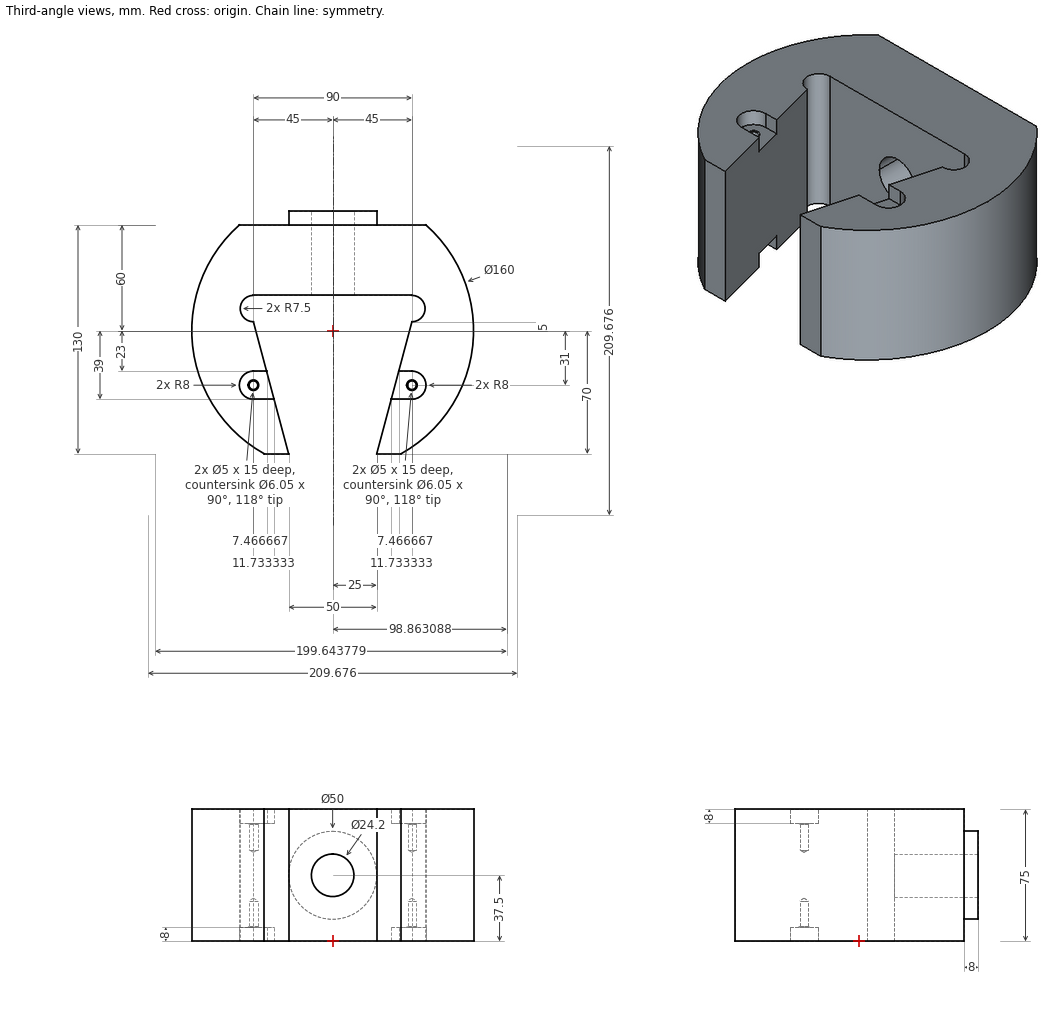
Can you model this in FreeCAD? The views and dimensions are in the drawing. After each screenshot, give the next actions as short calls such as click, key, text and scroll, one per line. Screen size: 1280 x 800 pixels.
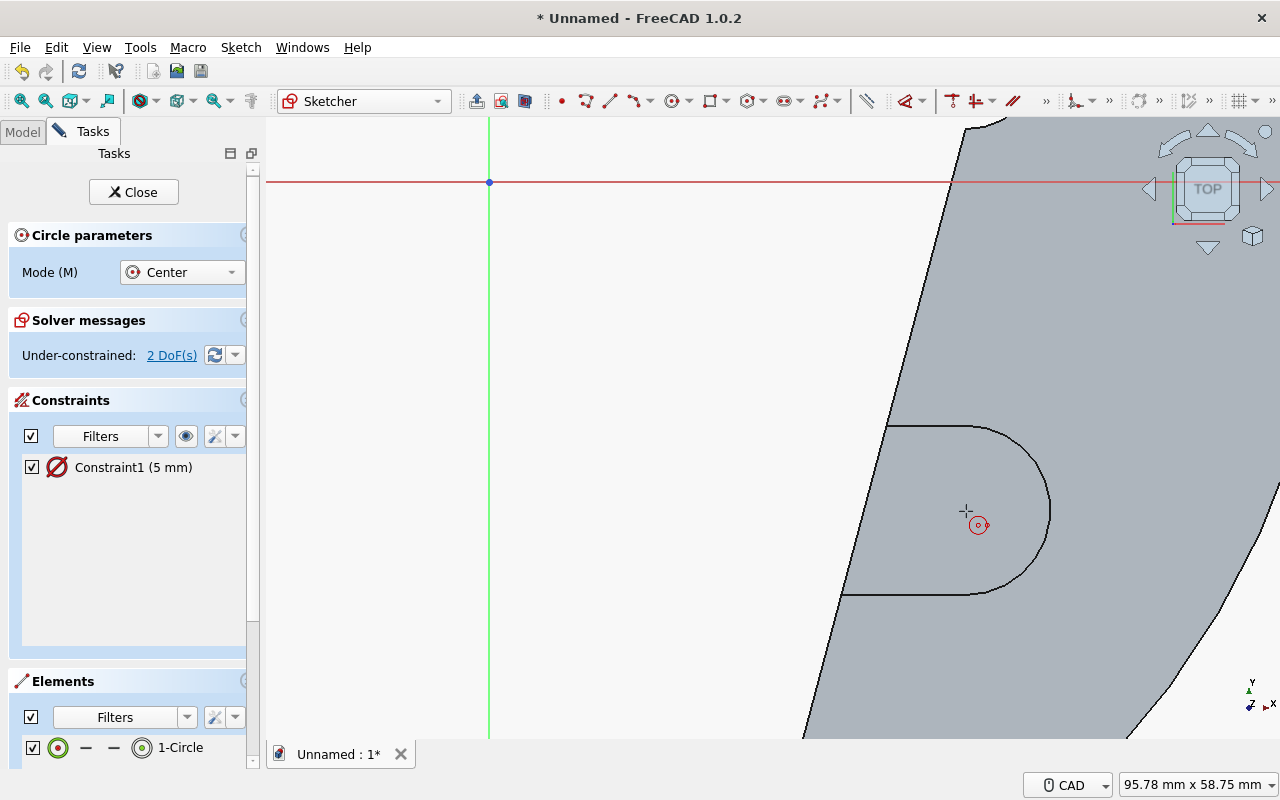
click(966, 510)
move(984, 492)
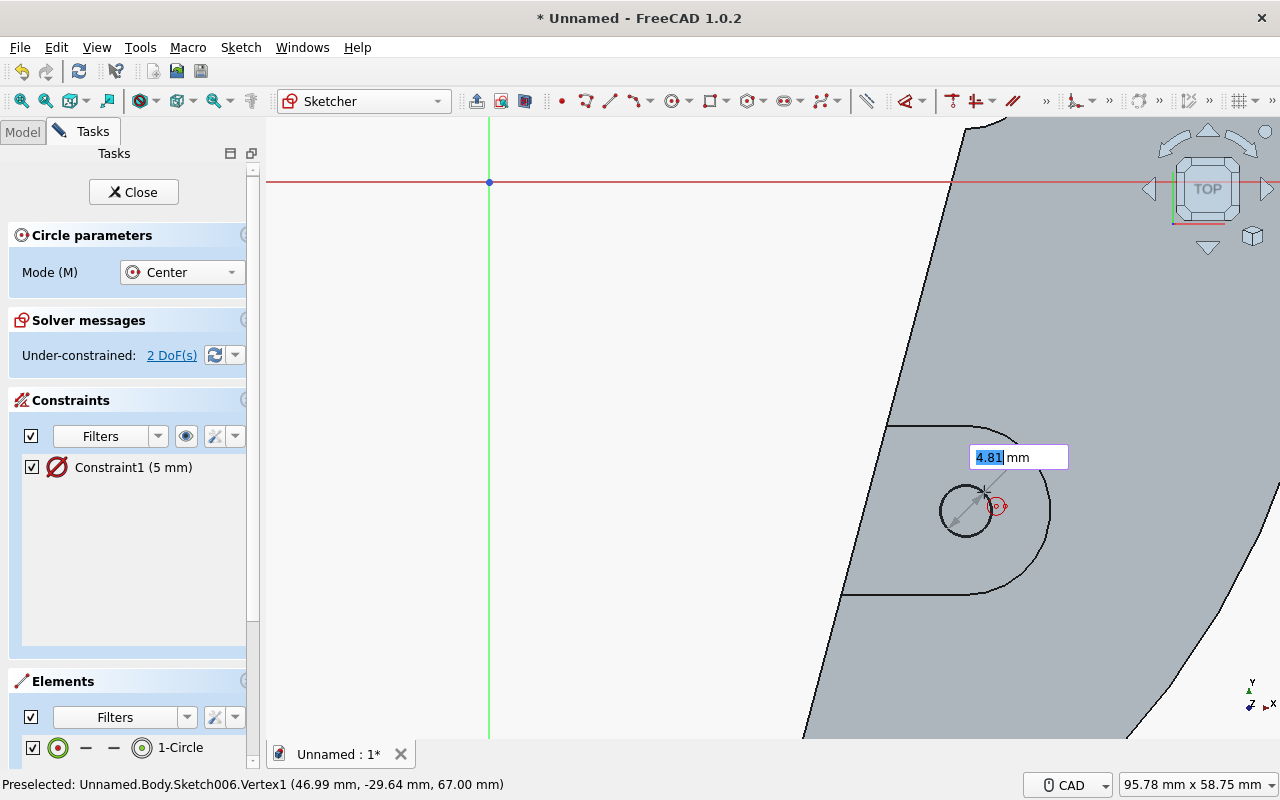
text(5)
key(Return)
key(Escape)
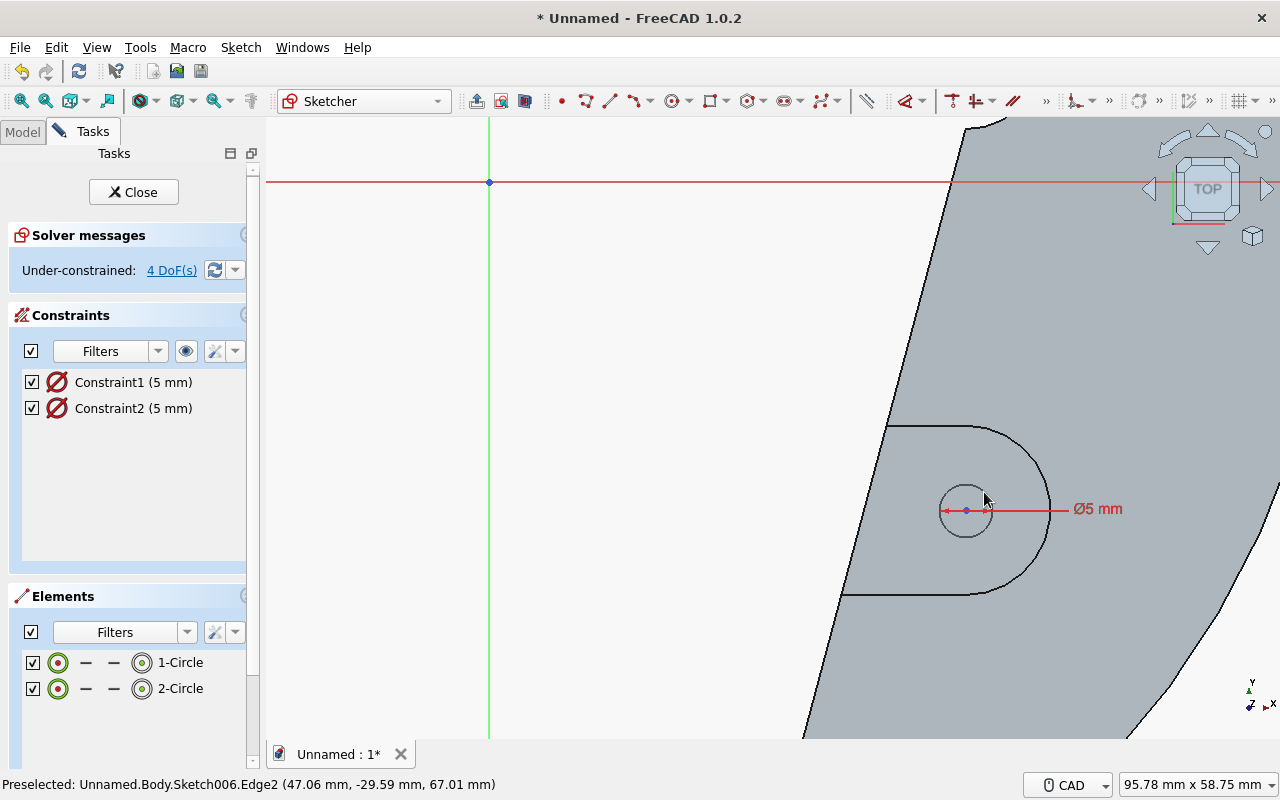
scroll(966, 511, down, 3)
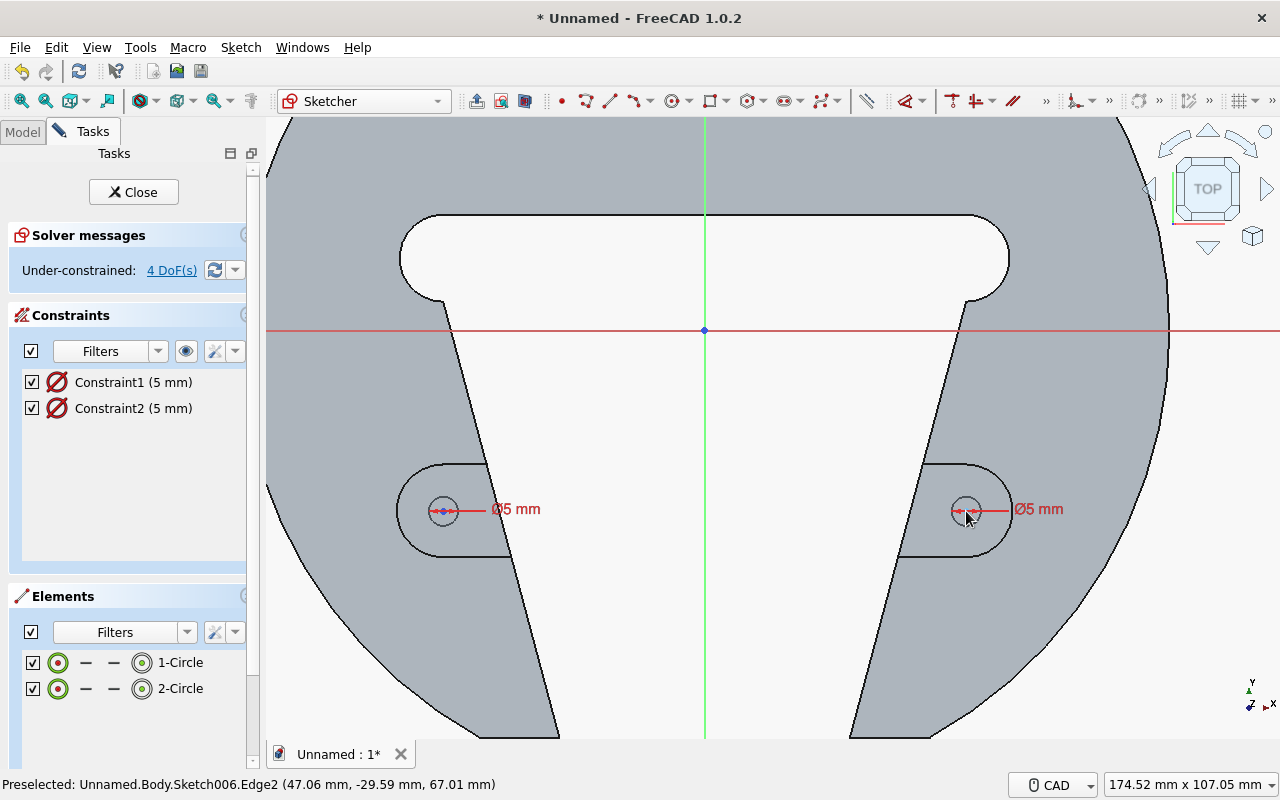
click(443, 511)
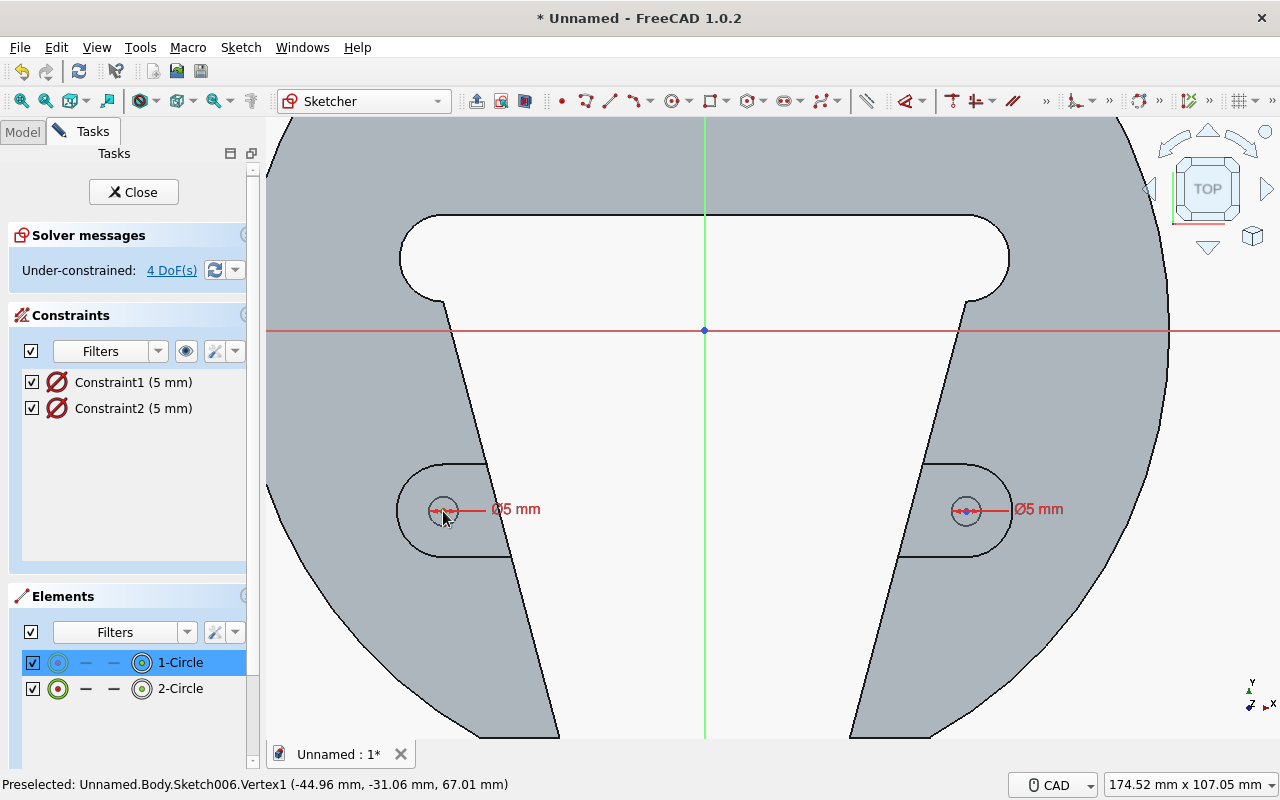
click(966, 511)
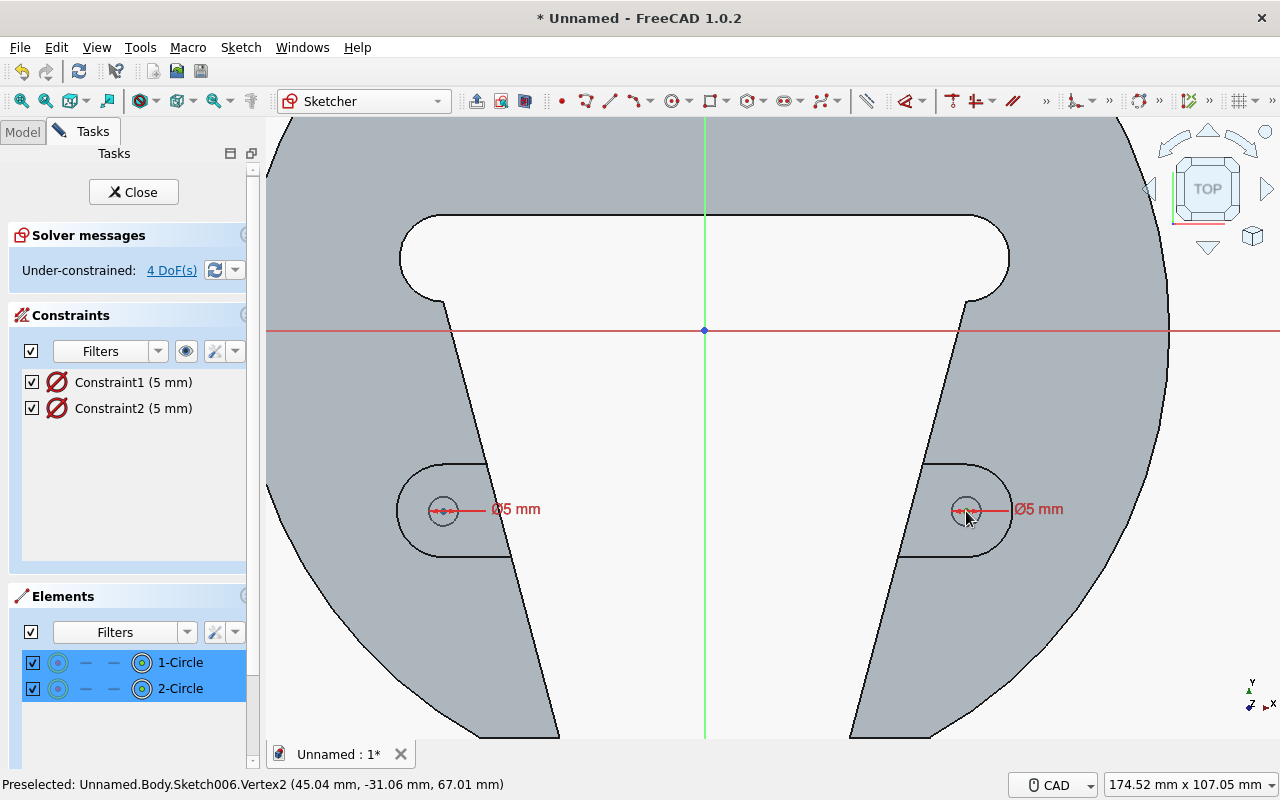
key(h)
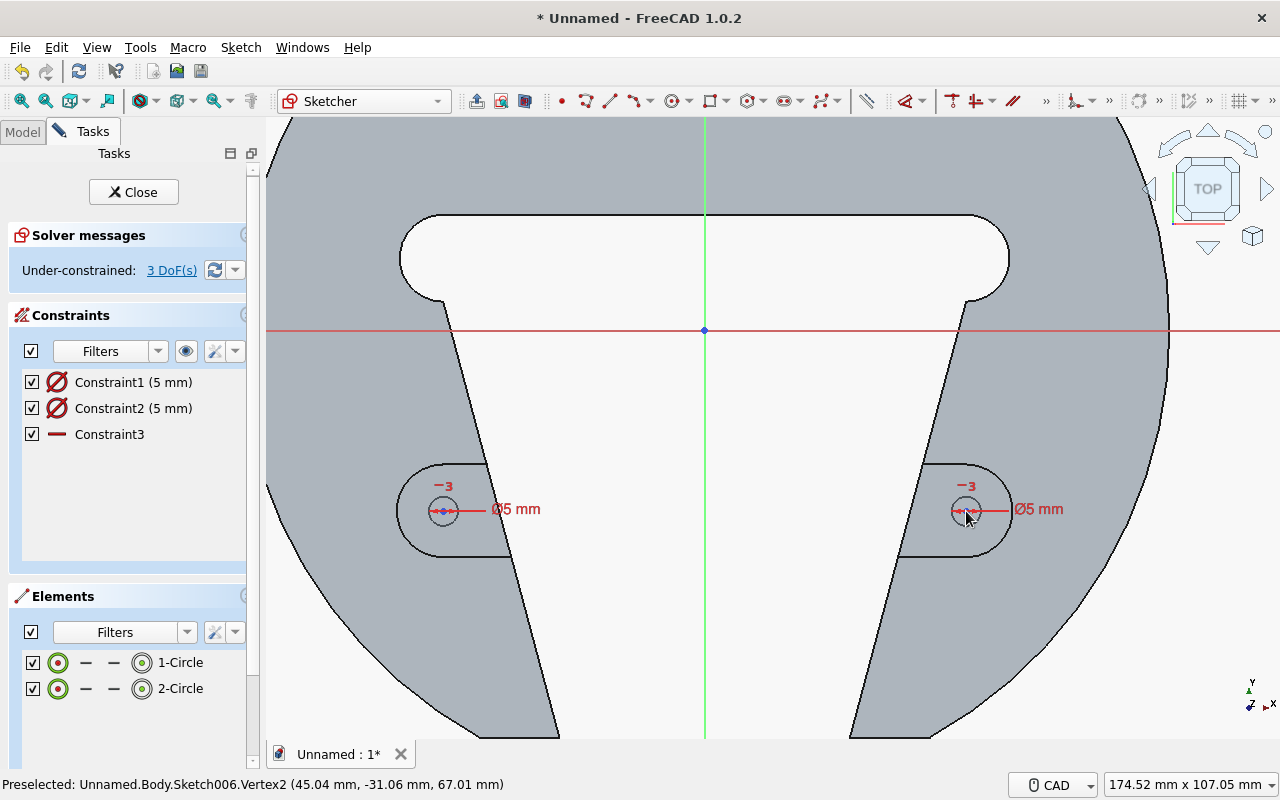
key(d)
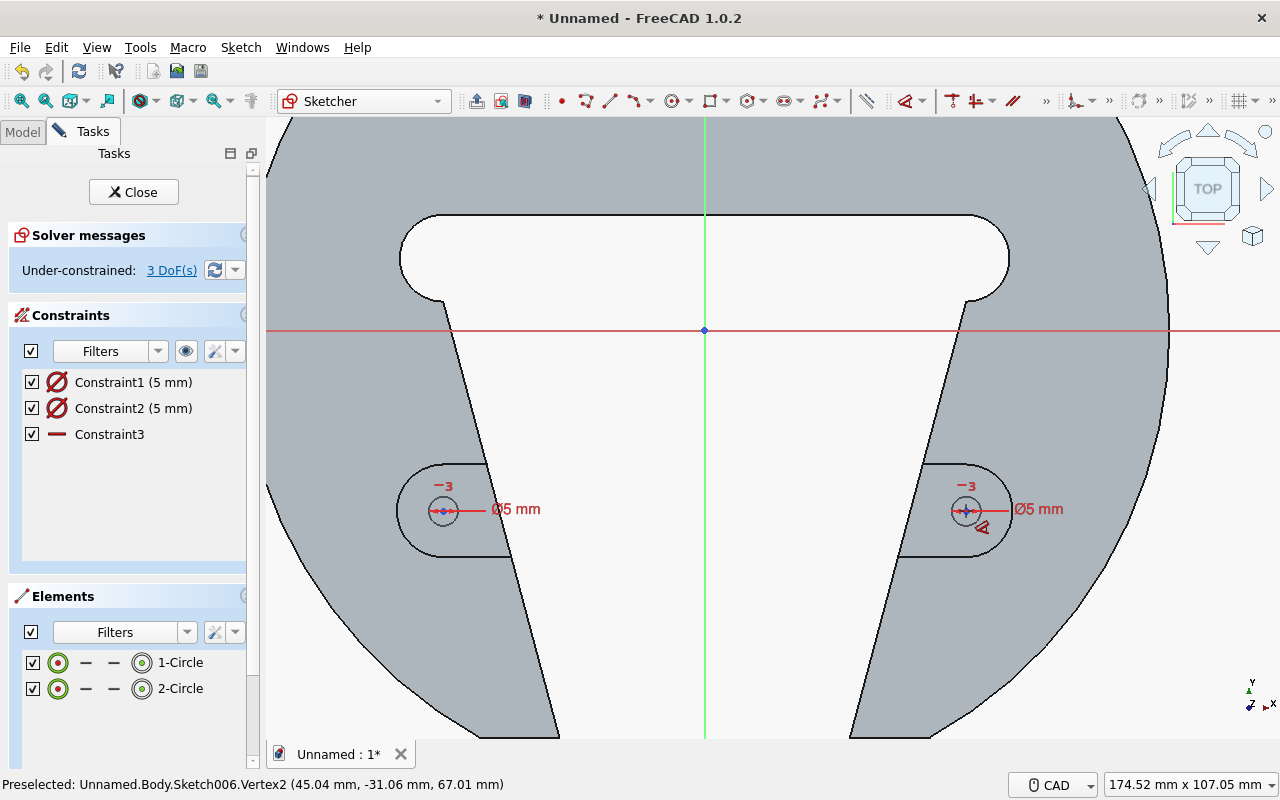
click(443, 511)
click(574, 297)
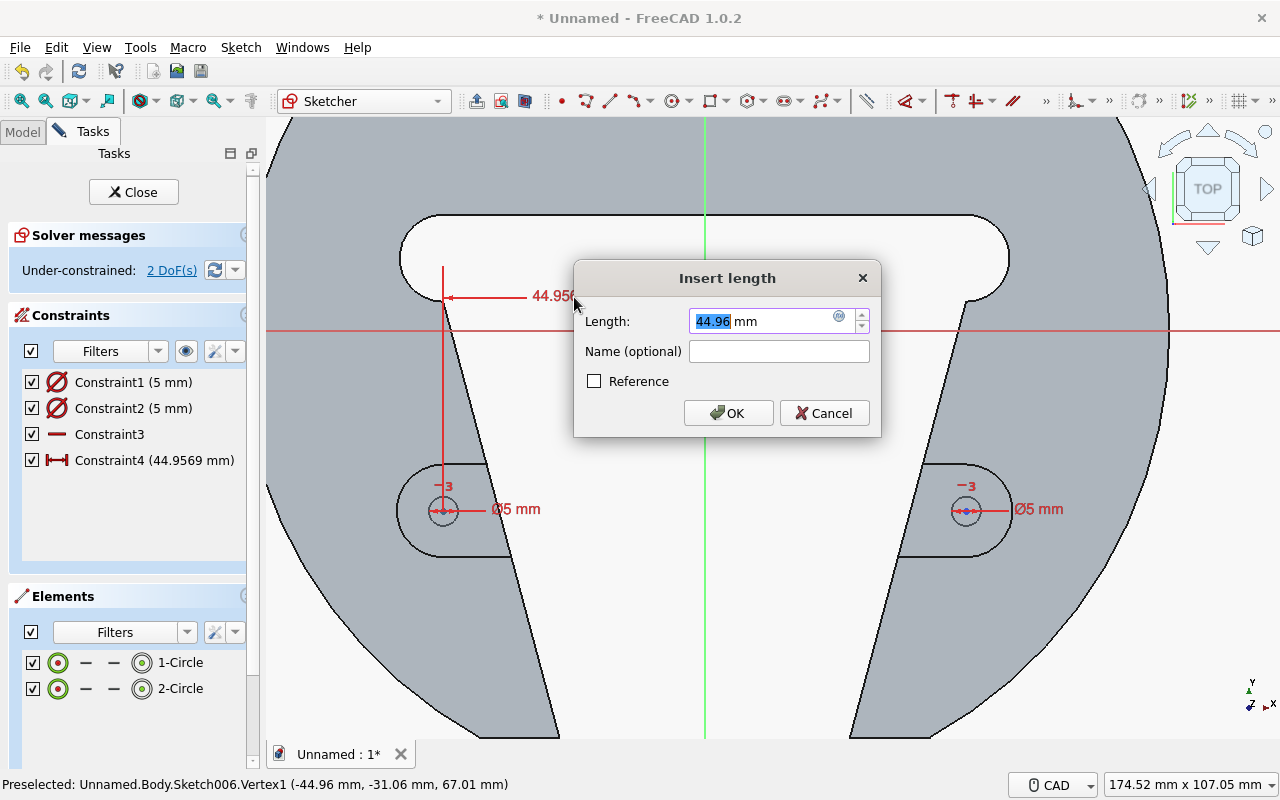
text(45)
key(Return)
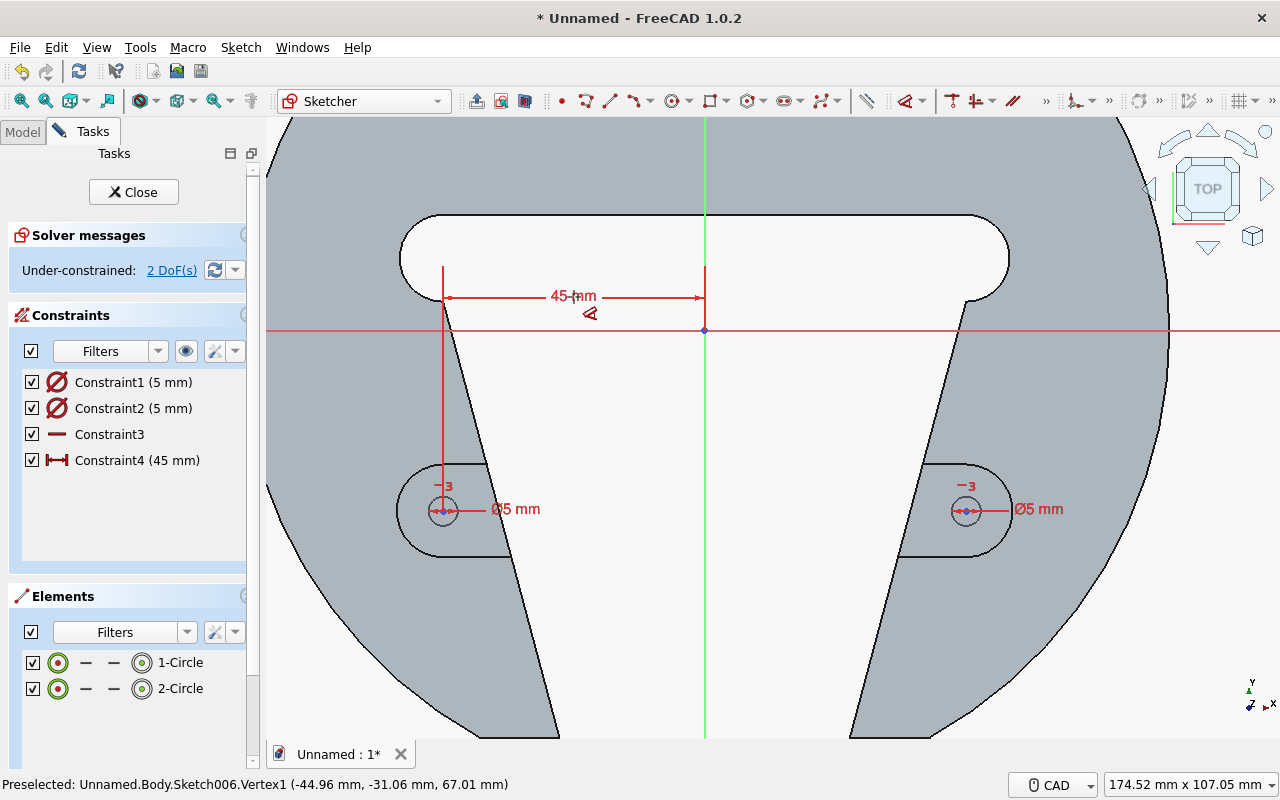
click(443, 511)
click(409, 421)